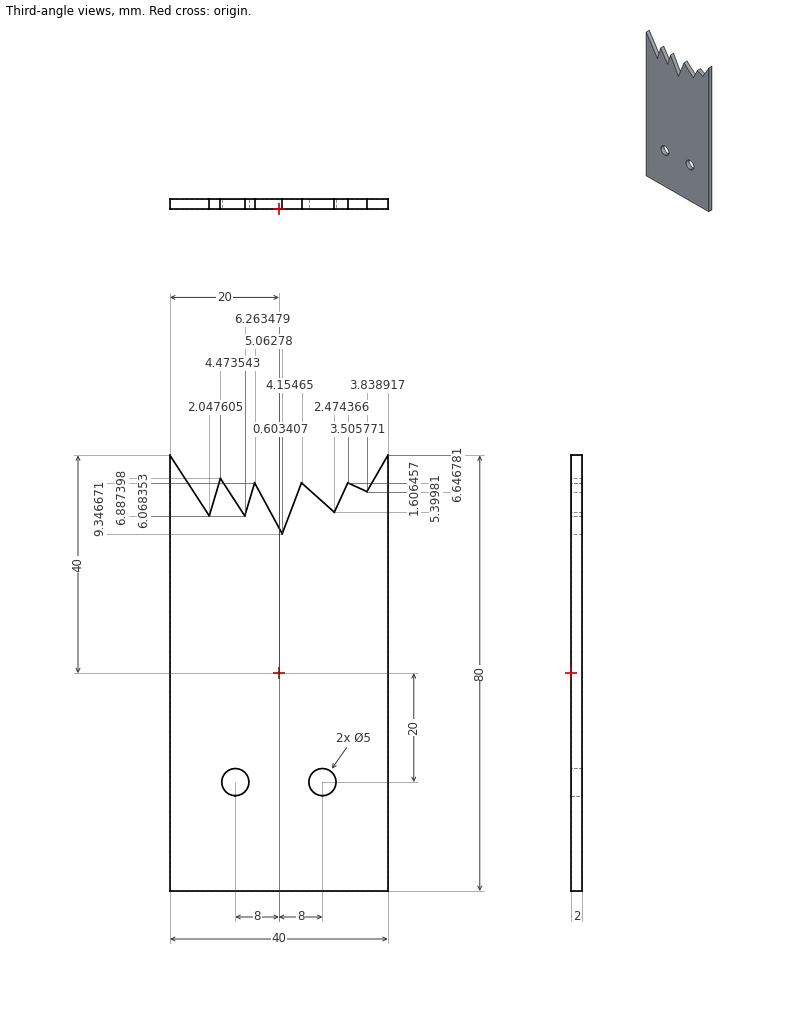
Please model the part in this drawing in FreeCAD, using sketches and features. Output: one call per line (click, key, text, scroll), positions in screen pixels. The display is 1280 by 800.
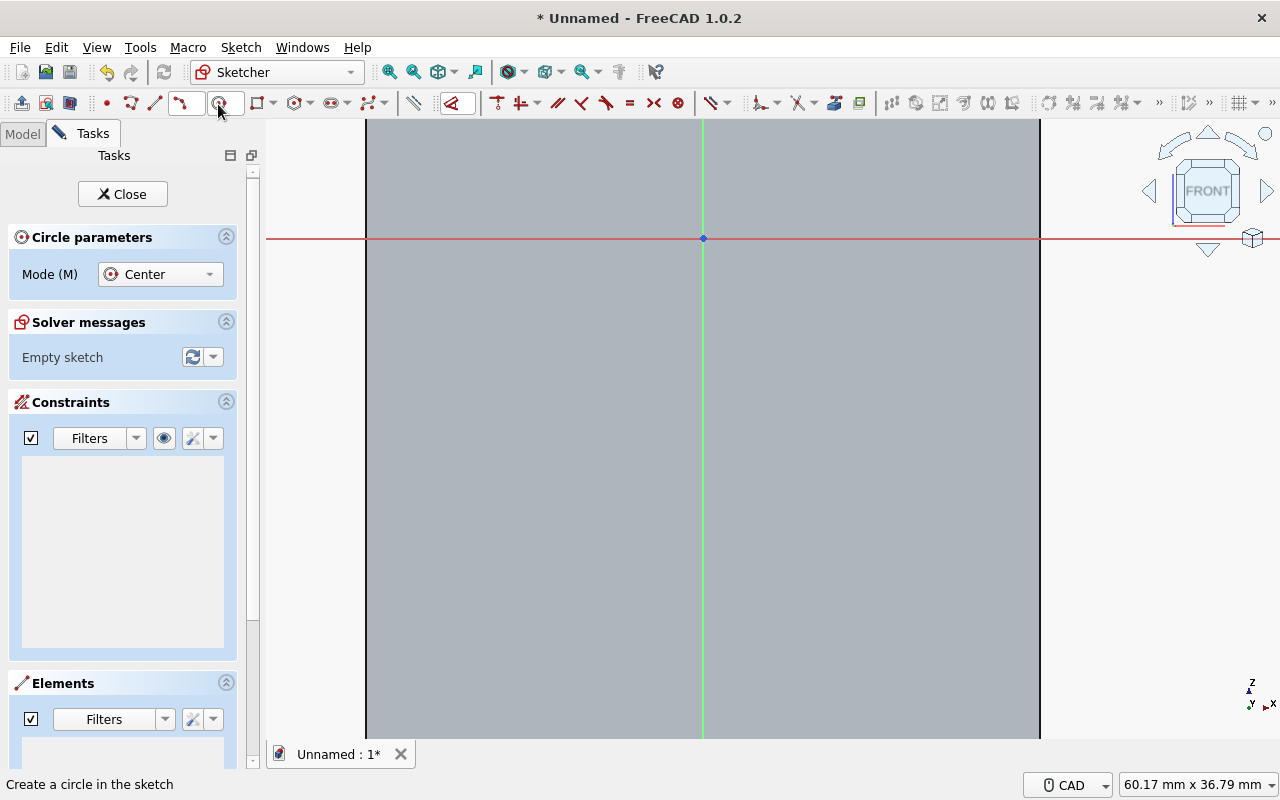
click(838, 576)
click(868, 546)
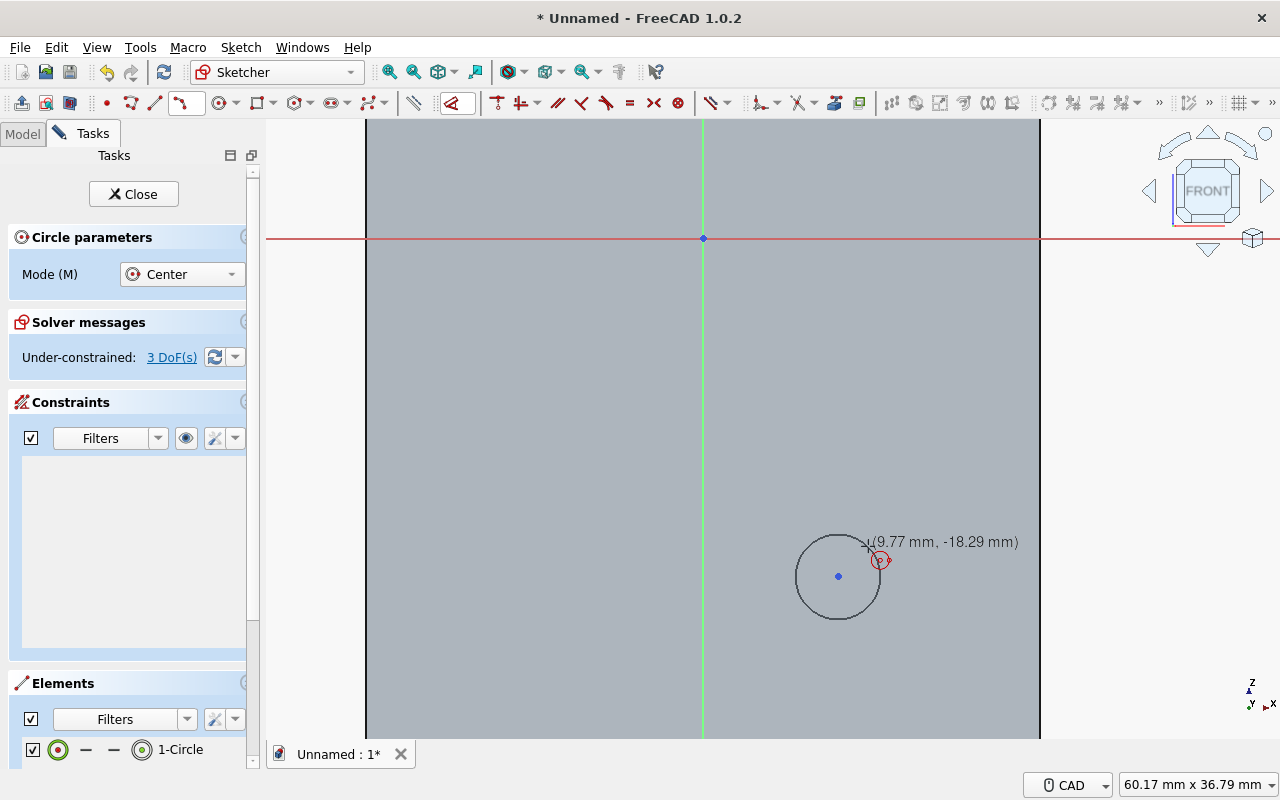
click(569, 576)
click(598, 546)
key(Escape)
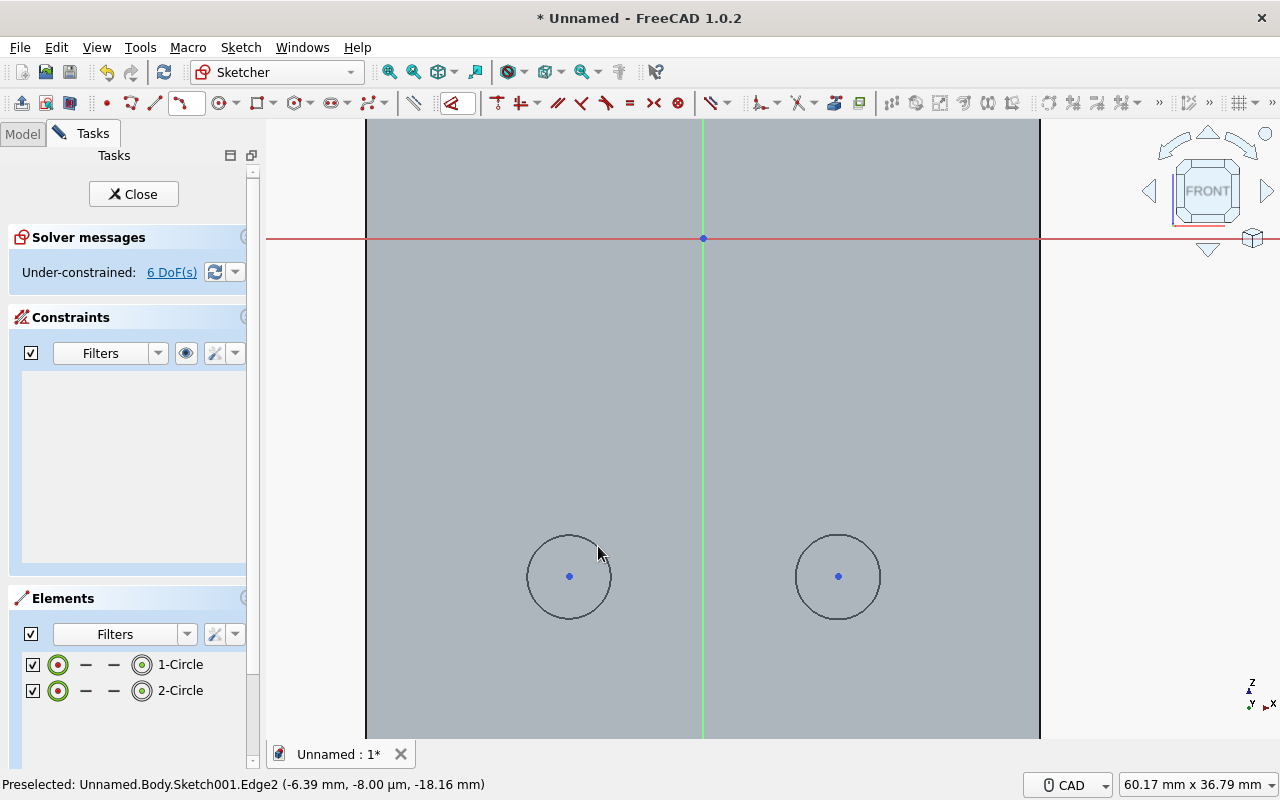
click(868, 547)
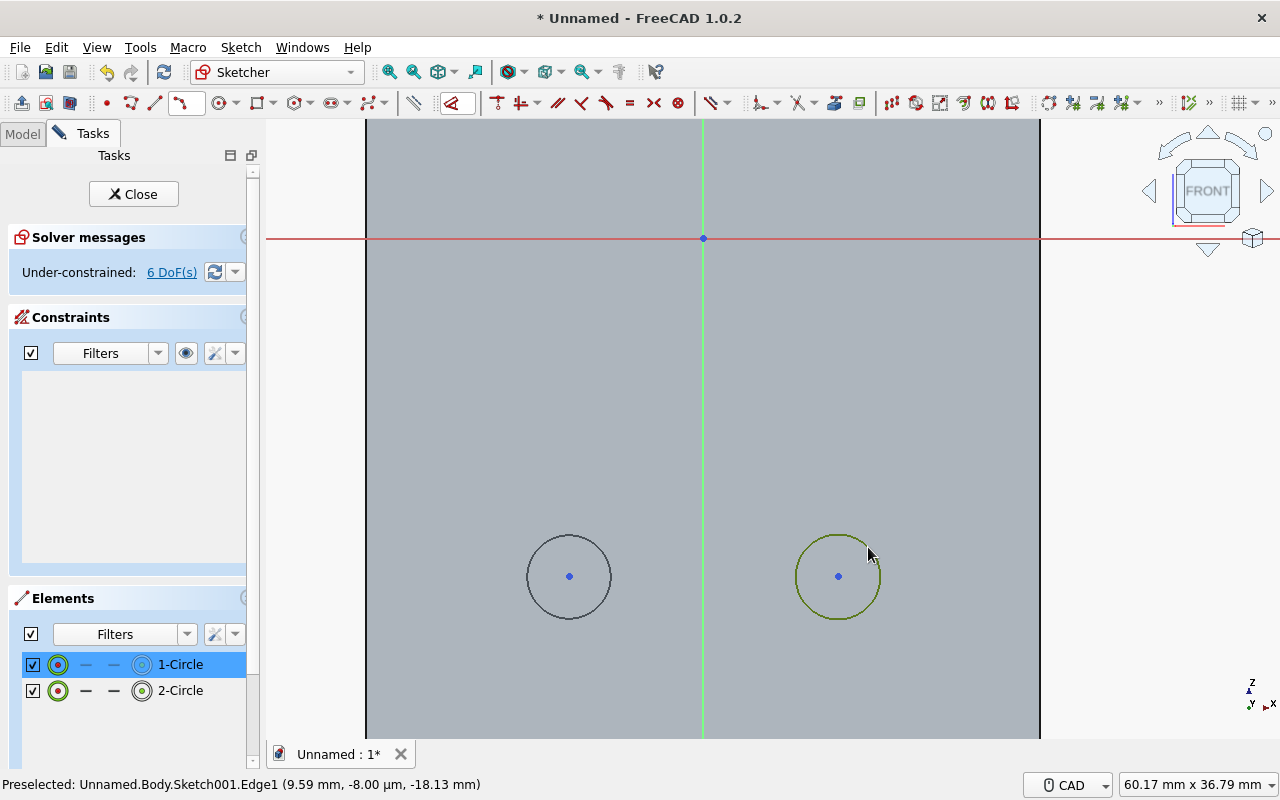
click(598, 547)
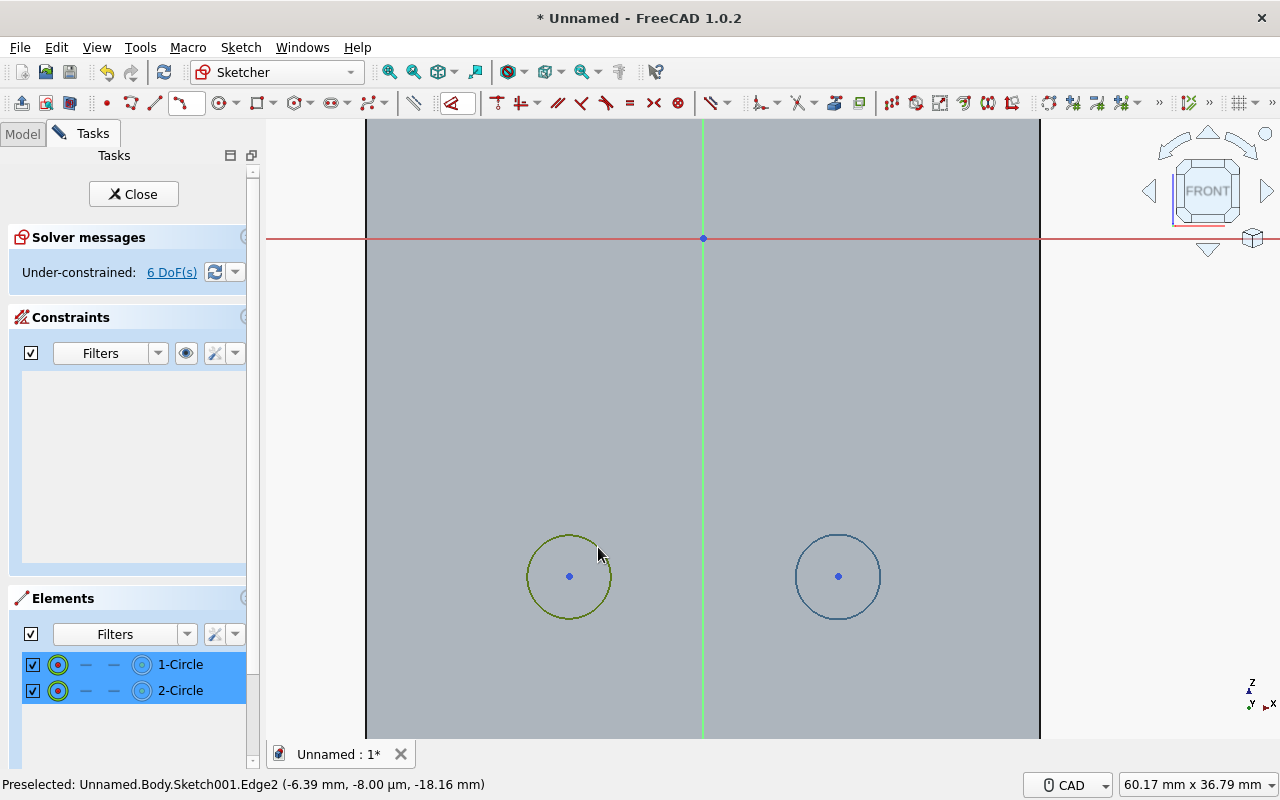
key(e)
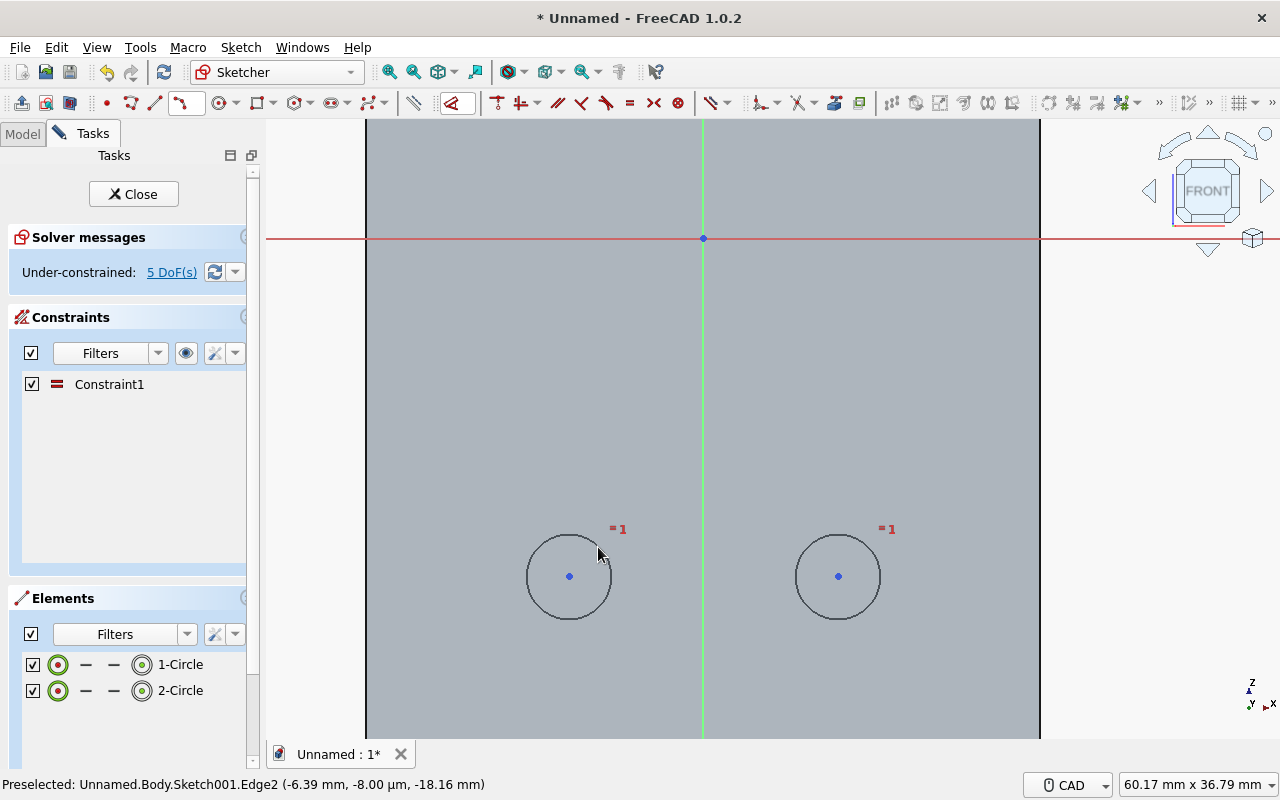
click(838, 577)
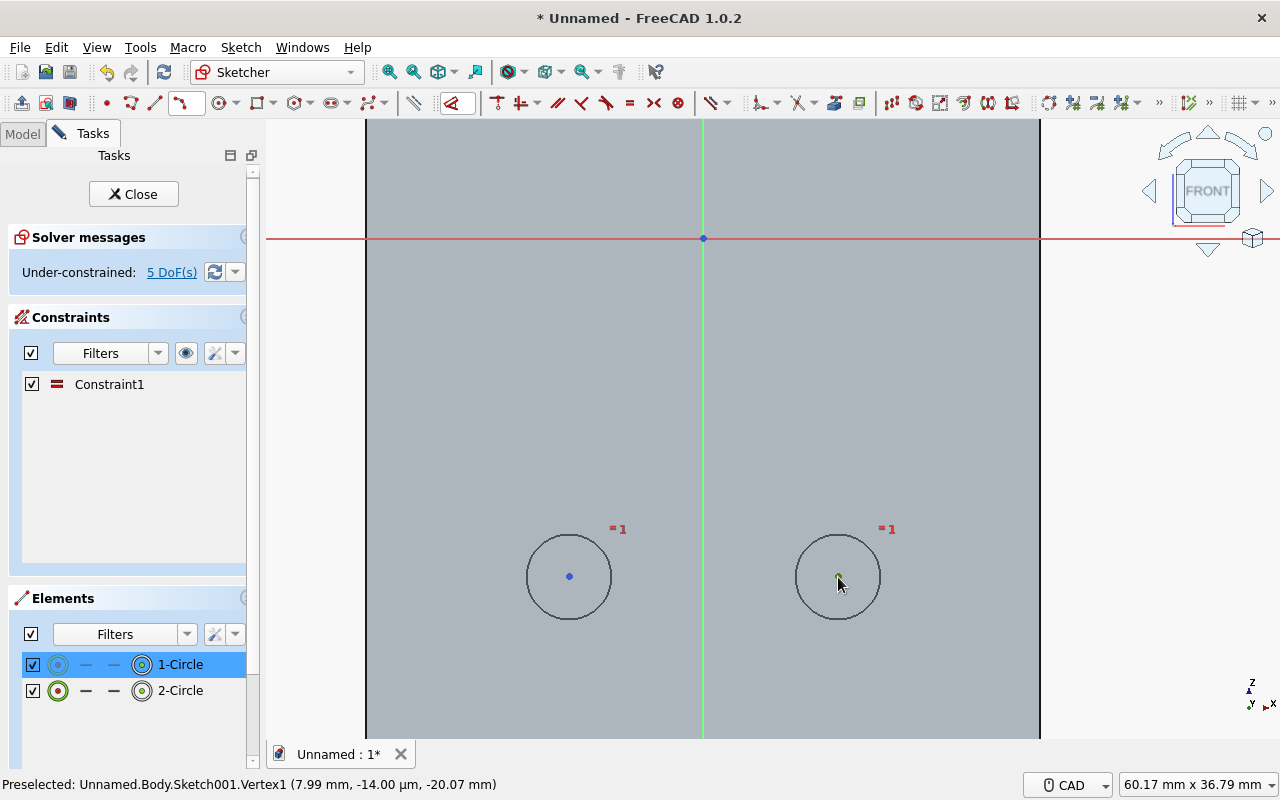
click(569, 577)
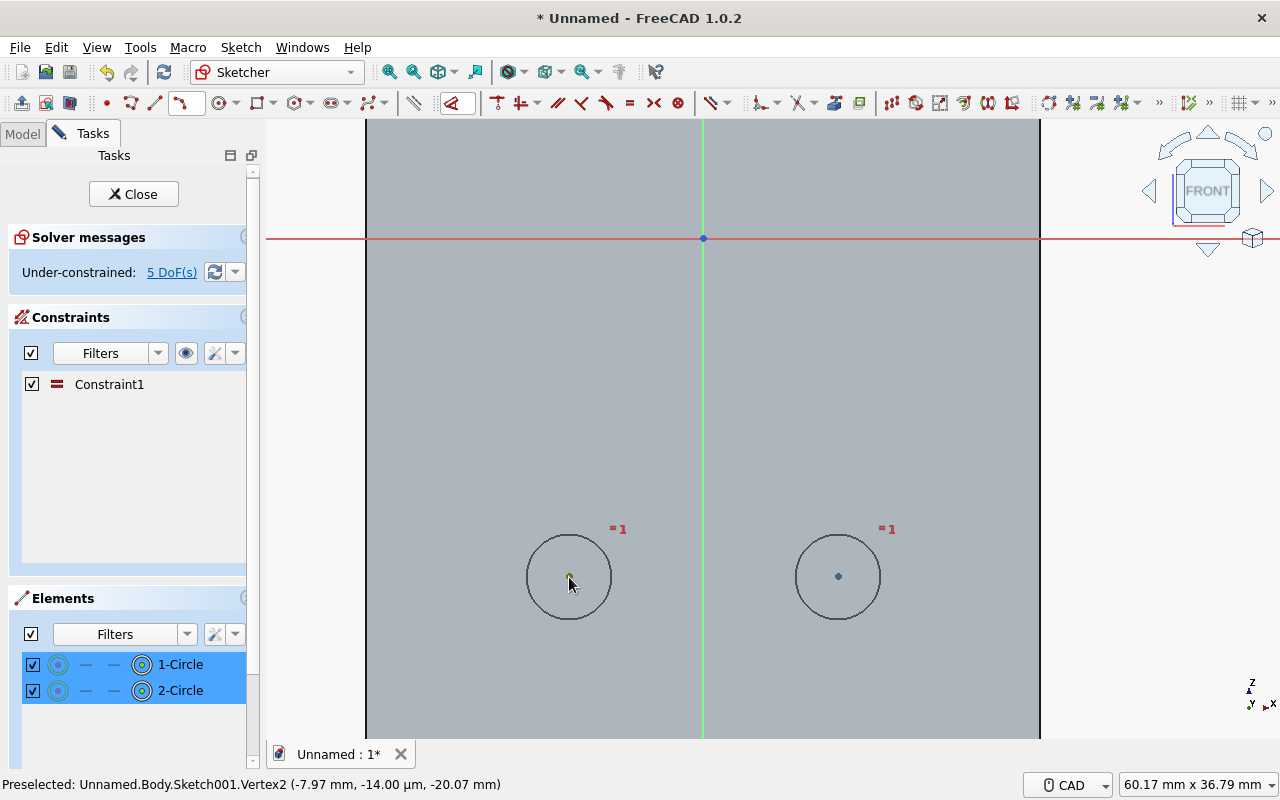
click(540, 104)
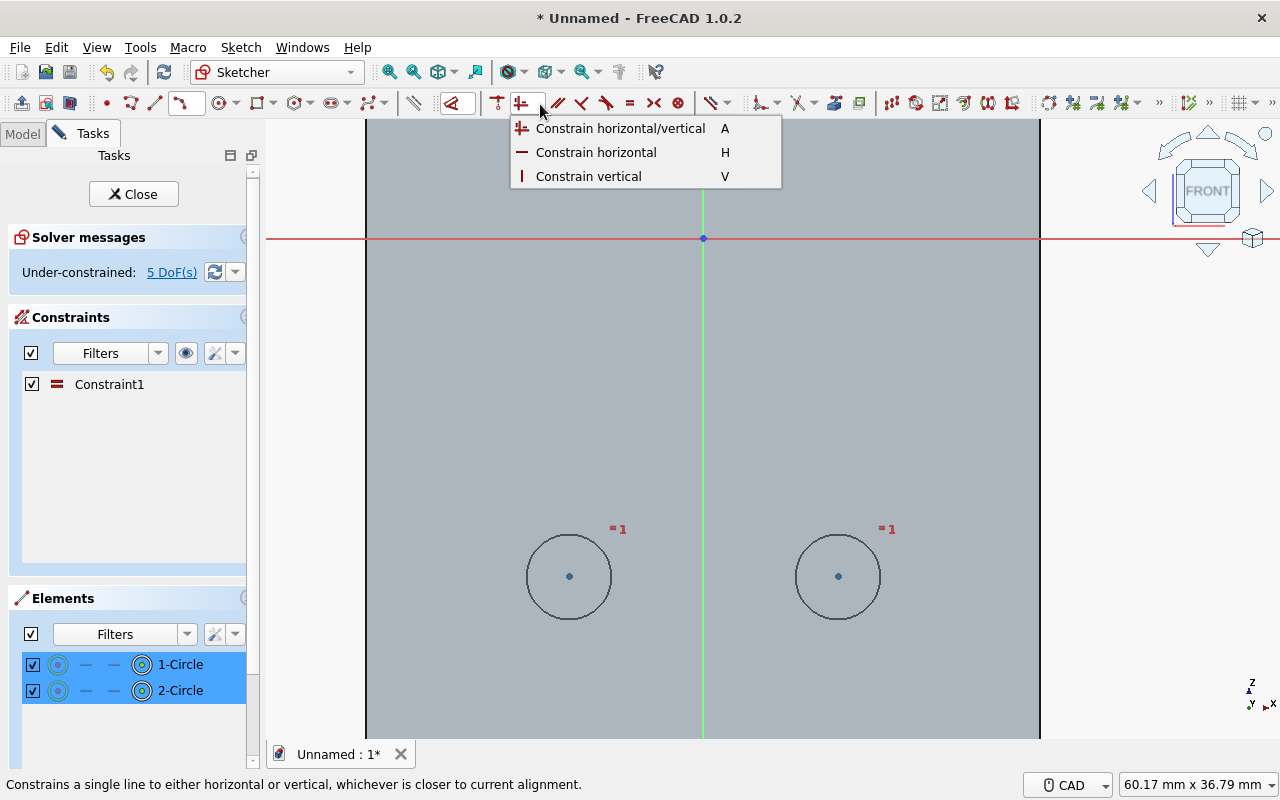
click(646, 152)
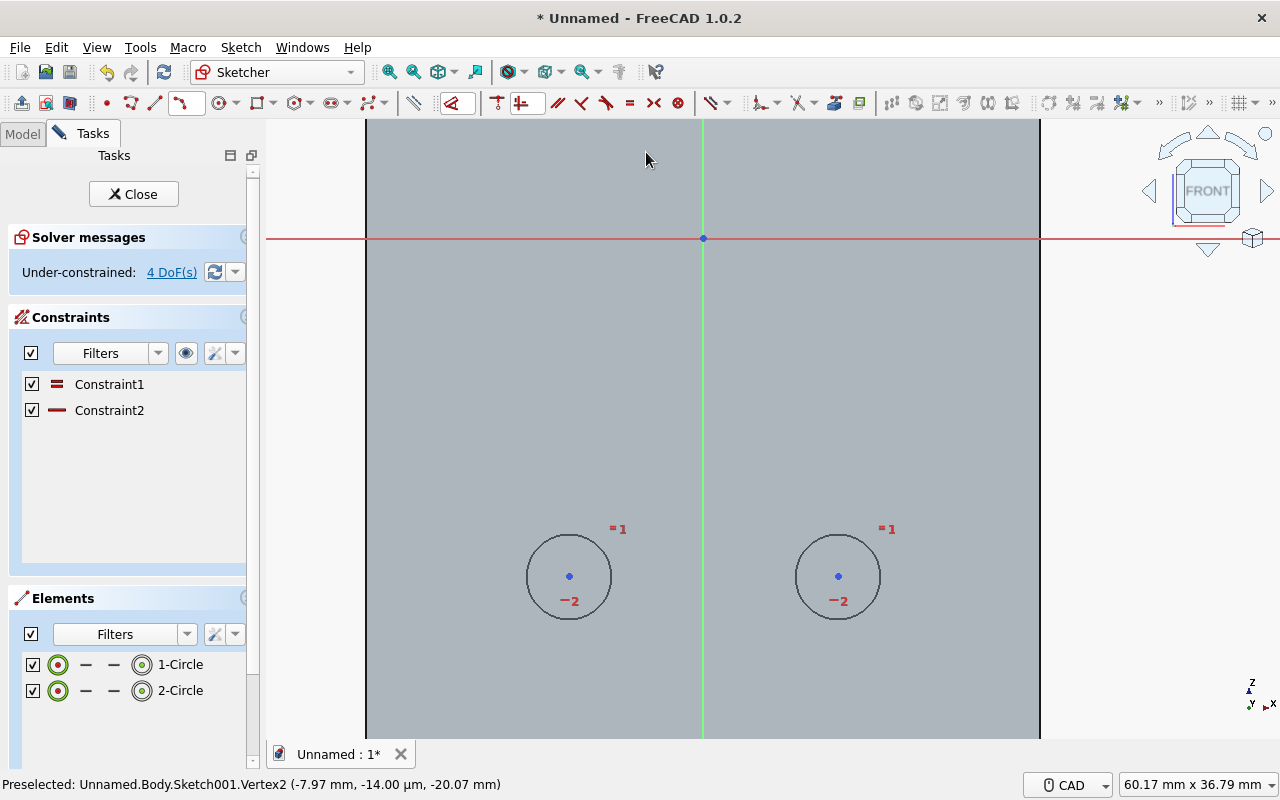
key(d)